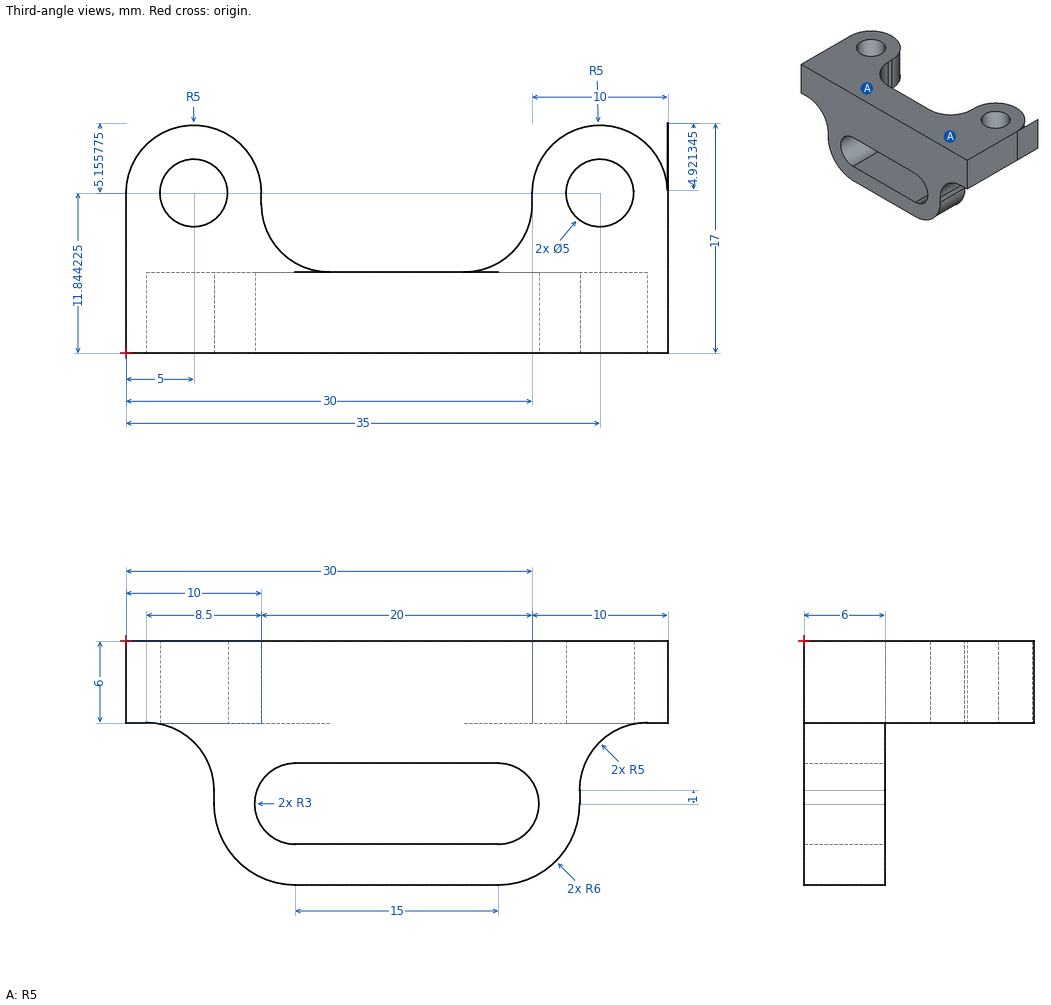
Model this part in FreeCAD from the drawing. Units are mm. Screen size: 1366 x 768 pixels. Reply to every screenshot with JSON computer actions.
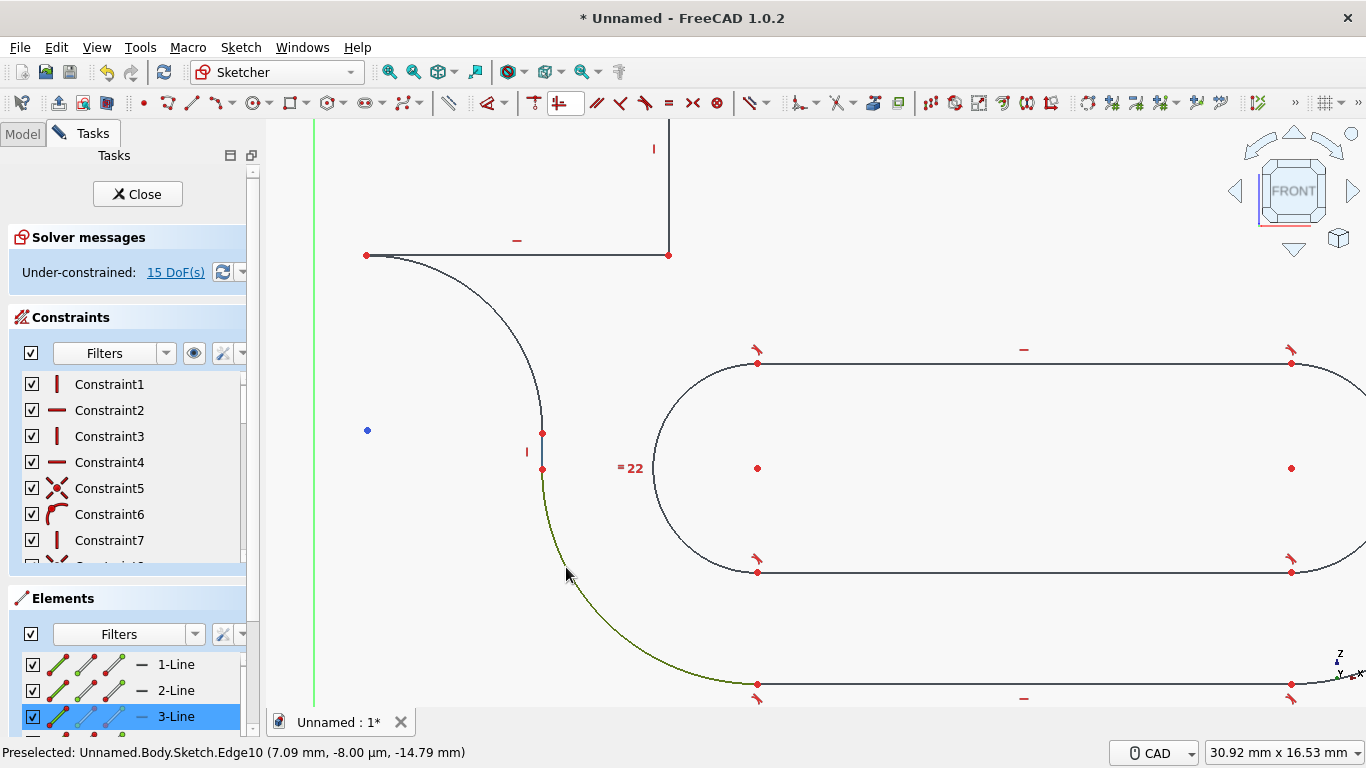
{"action": "key", "text": "t"}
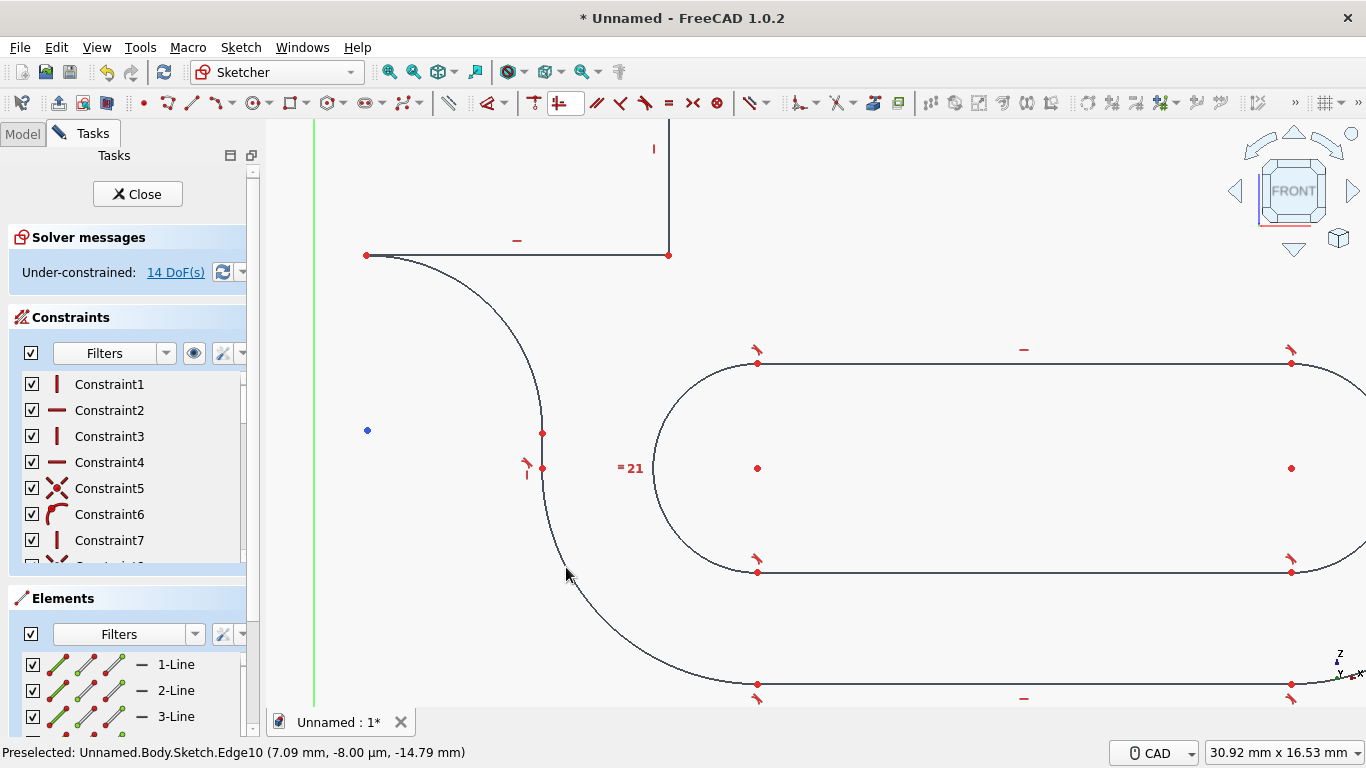
{"action": "scroll", "coordinate": [542, 458], "scroll_direction": "up", "scroll_amount": 2}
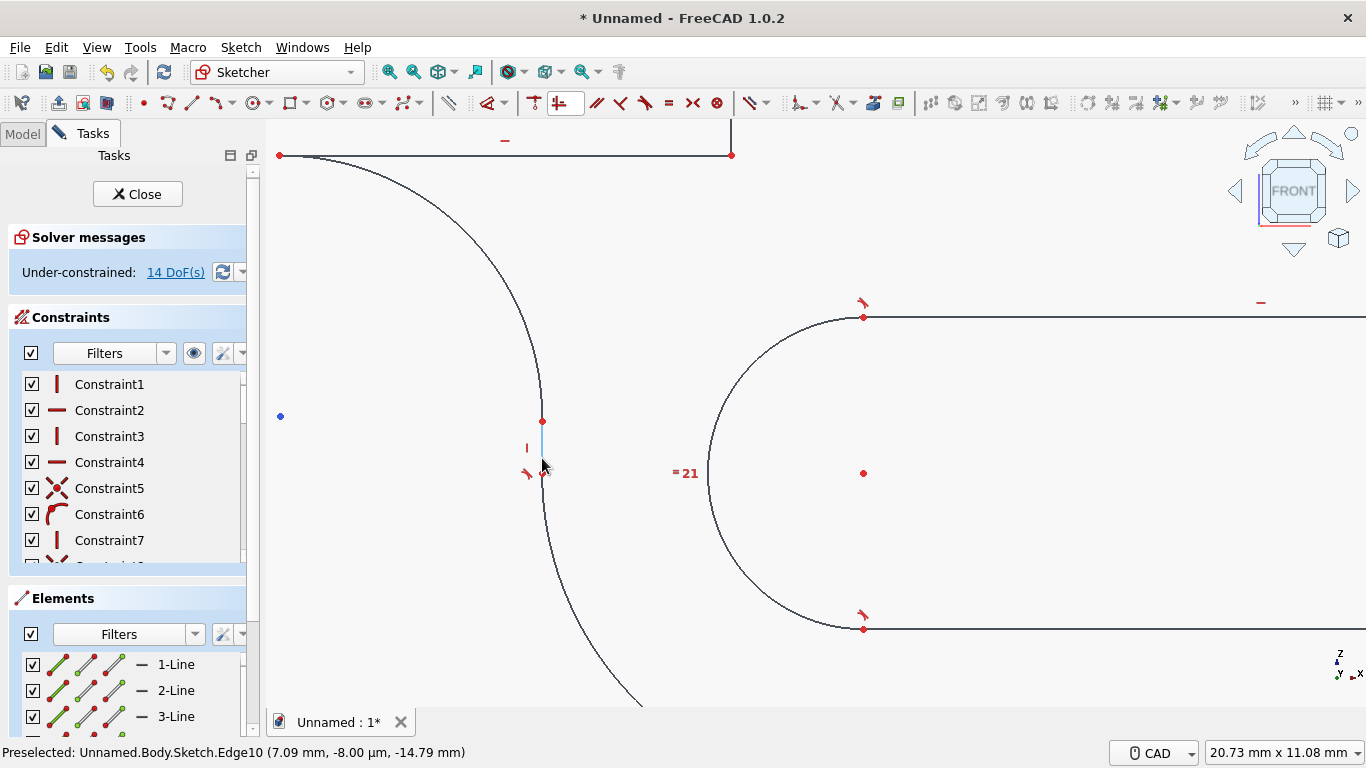
{"action": "left_click", "coordinate": [542, 458]}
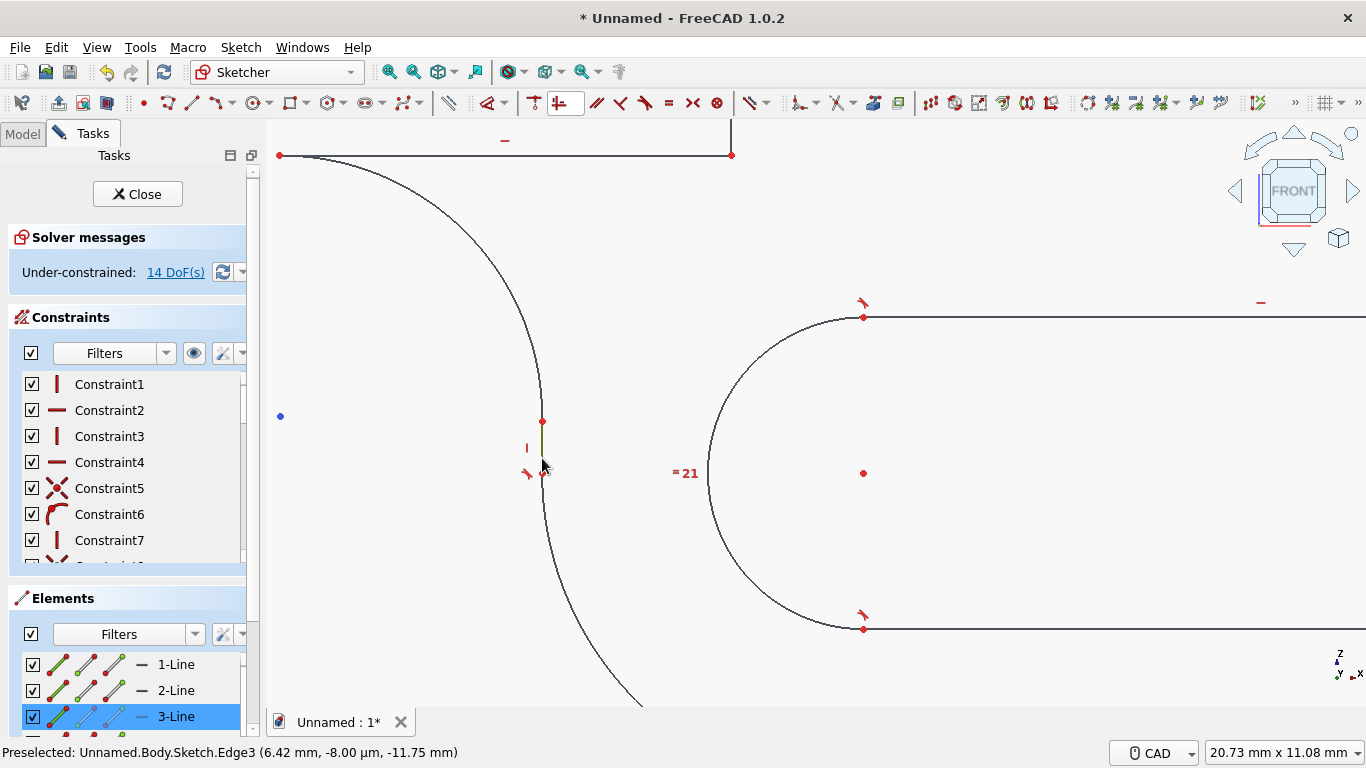
{"action": "left_click", "coordinate": [515, 301]}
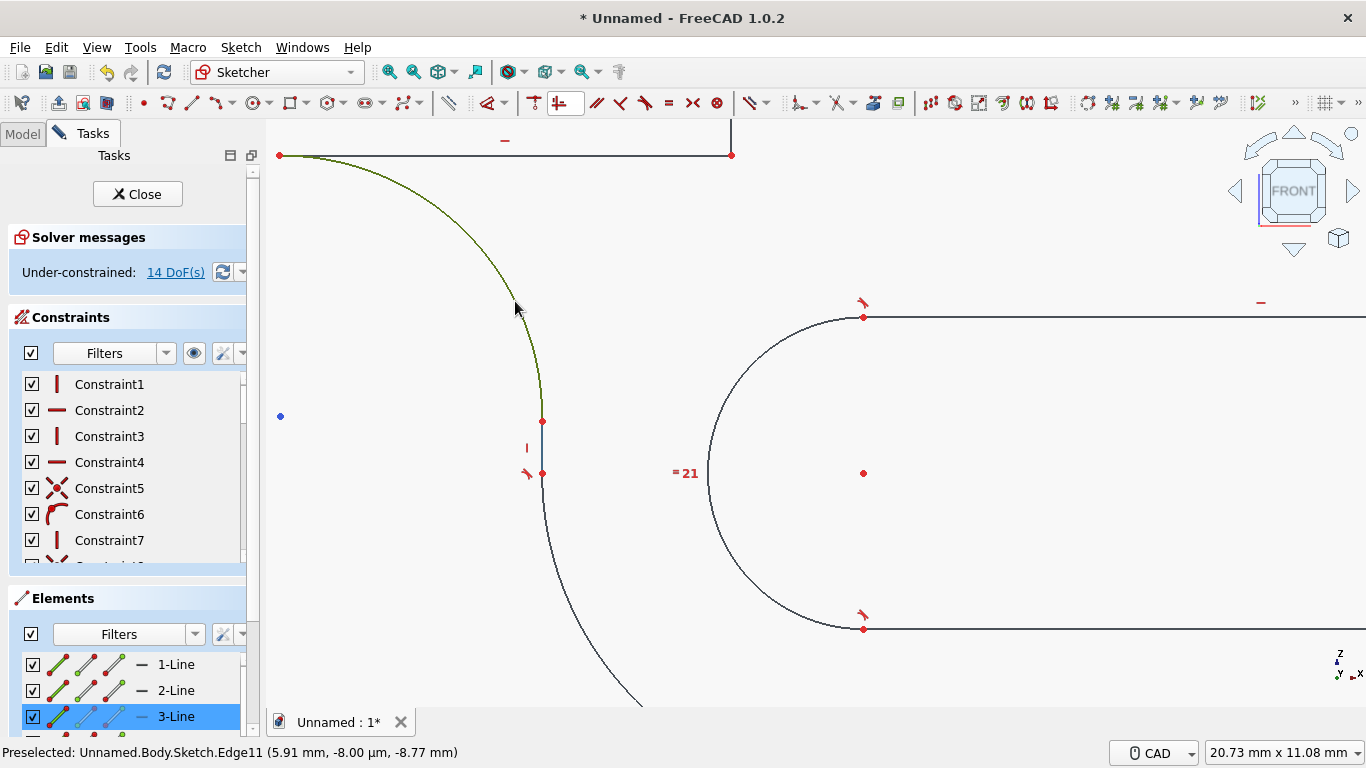
{"action": "key", "text": "t"}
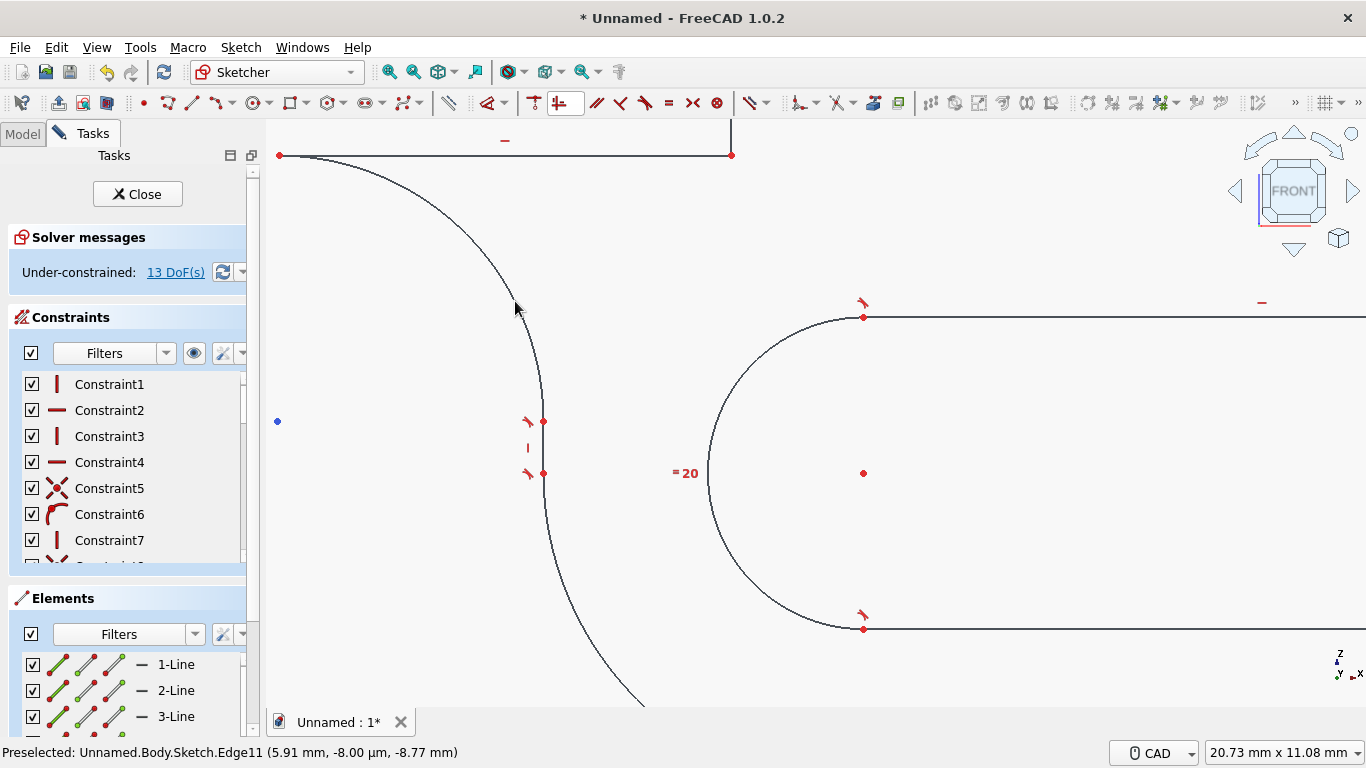
{"action": "left_click", "coordinate": [415, 156]}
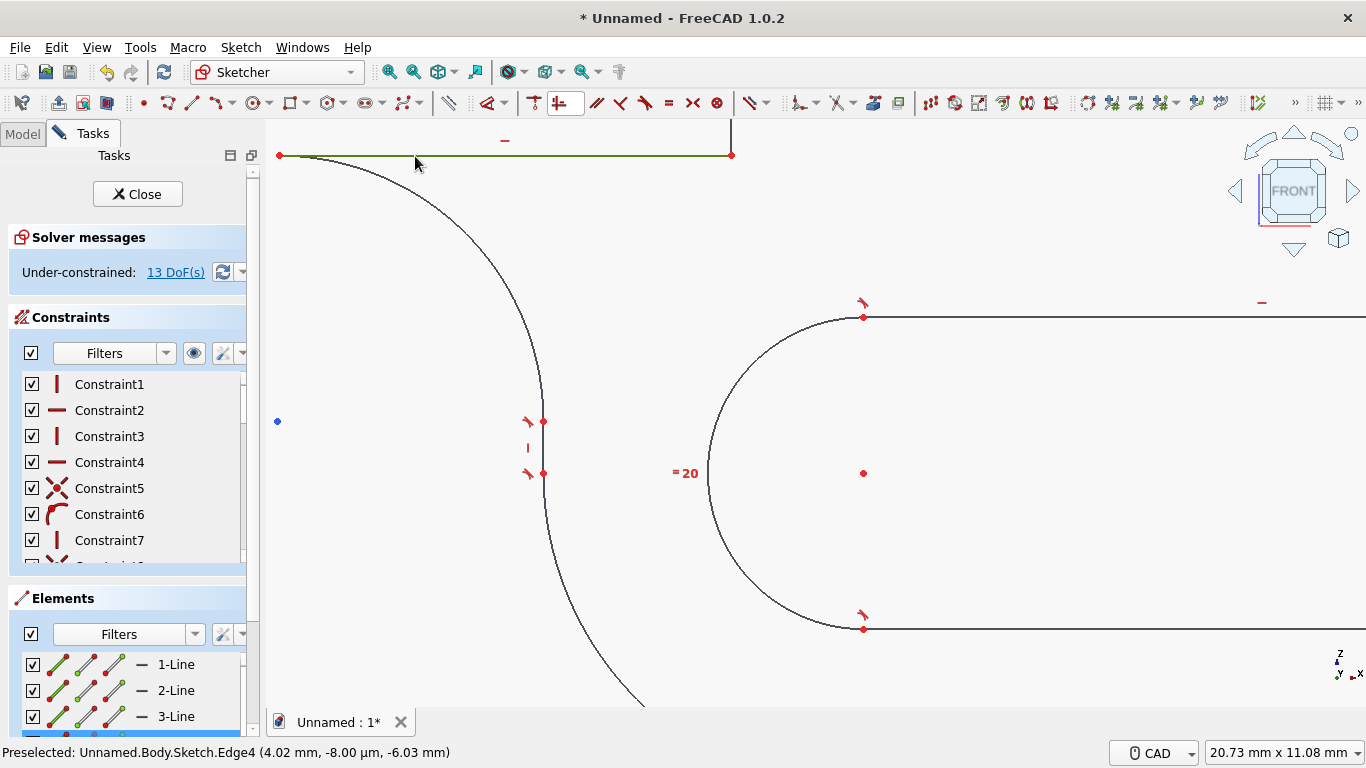
{"action": "left_click", "coordinate": [515, 301]}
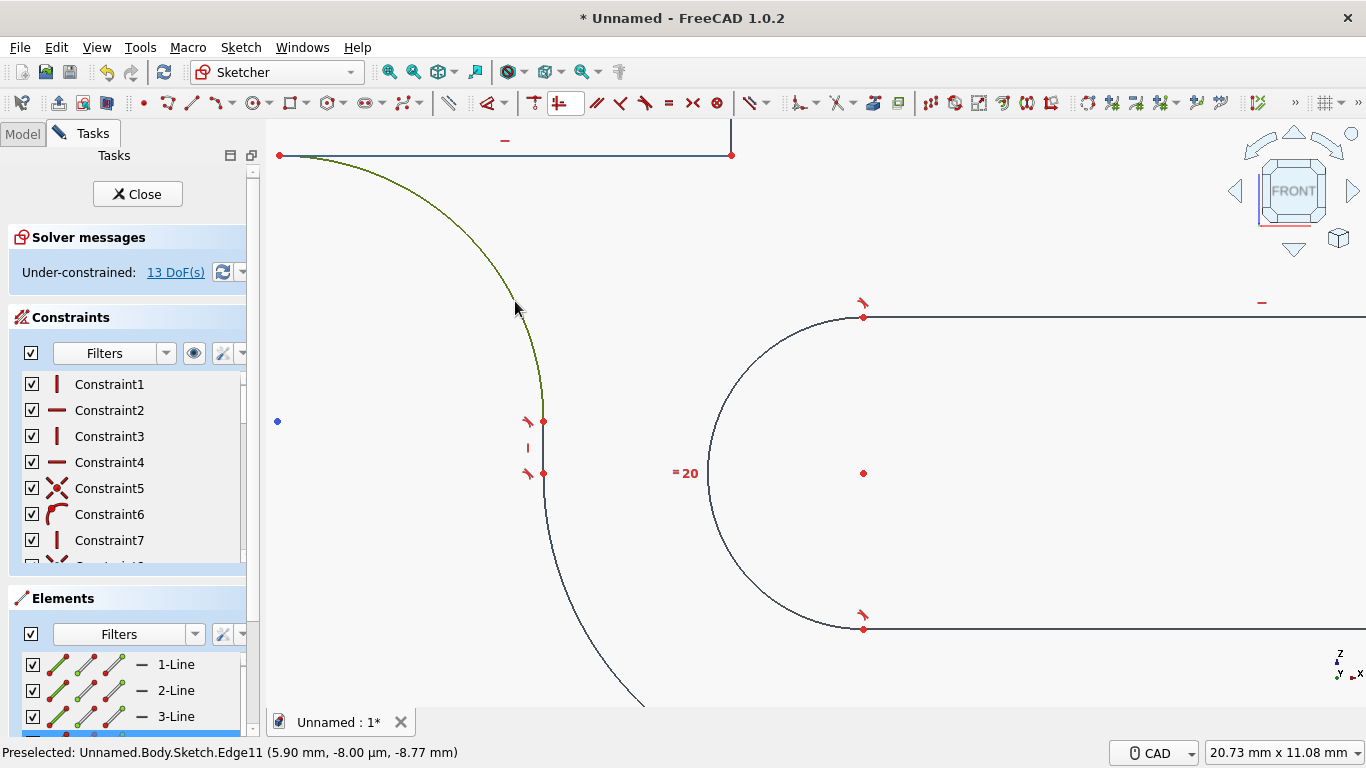
{"action": "left_click", "coordinate": [646, 104]}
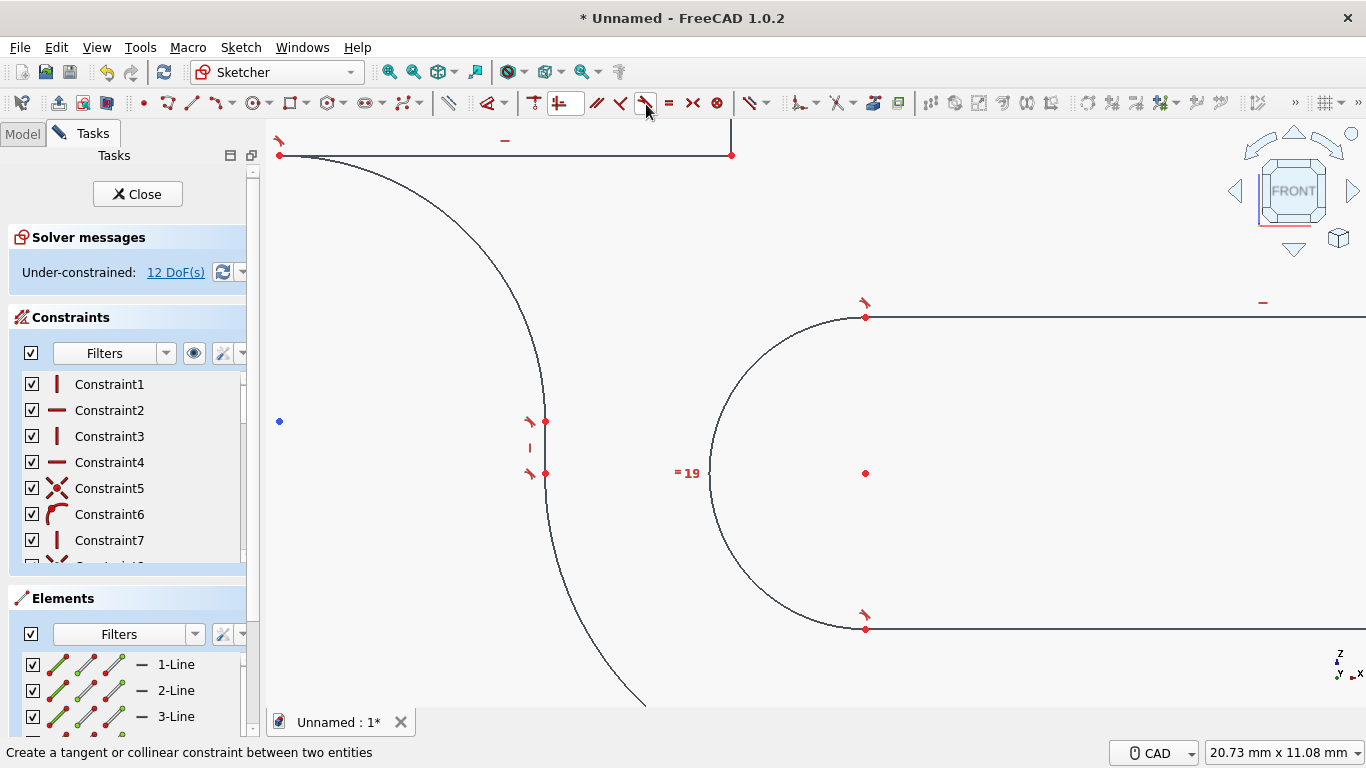
{"action": "scroll", "coordinate": [543, 456], "scroll_direction": "down", "scroll_amount": 6}